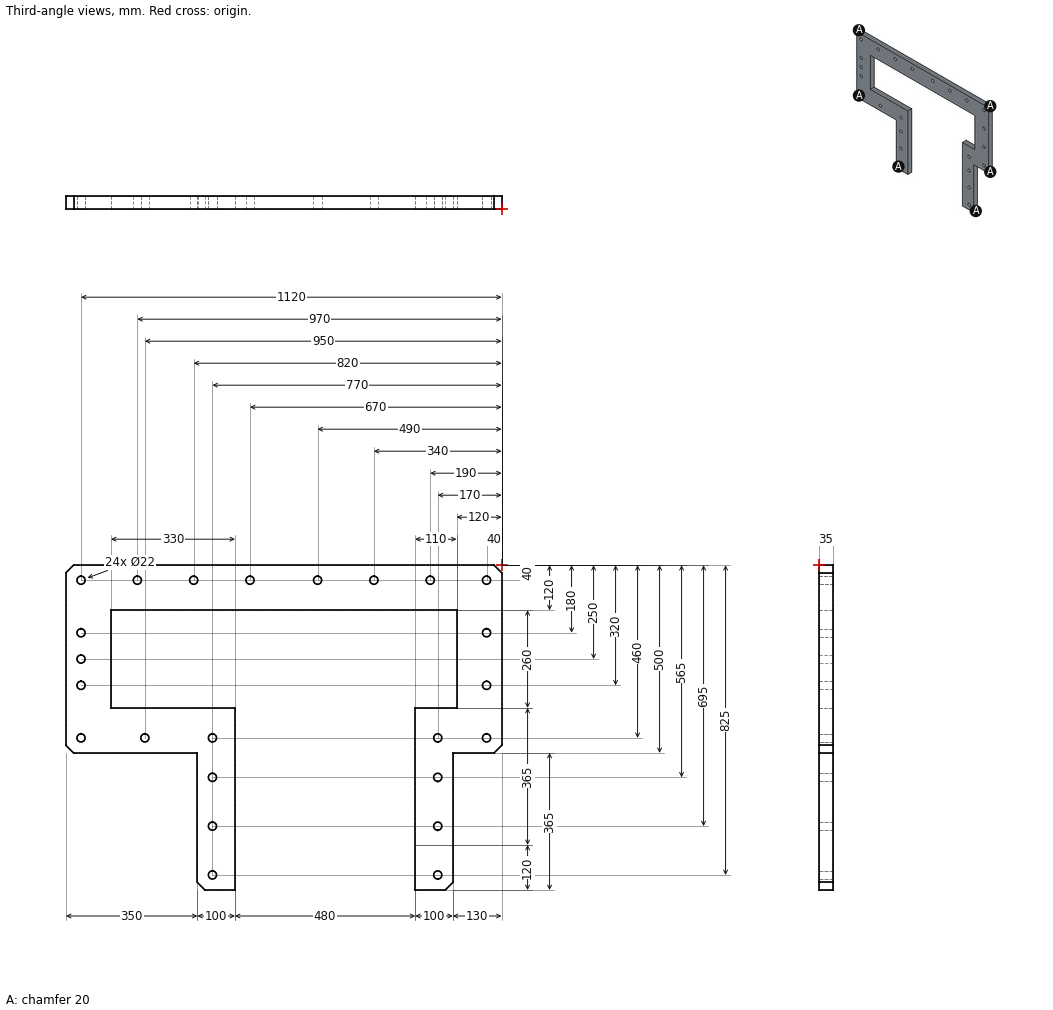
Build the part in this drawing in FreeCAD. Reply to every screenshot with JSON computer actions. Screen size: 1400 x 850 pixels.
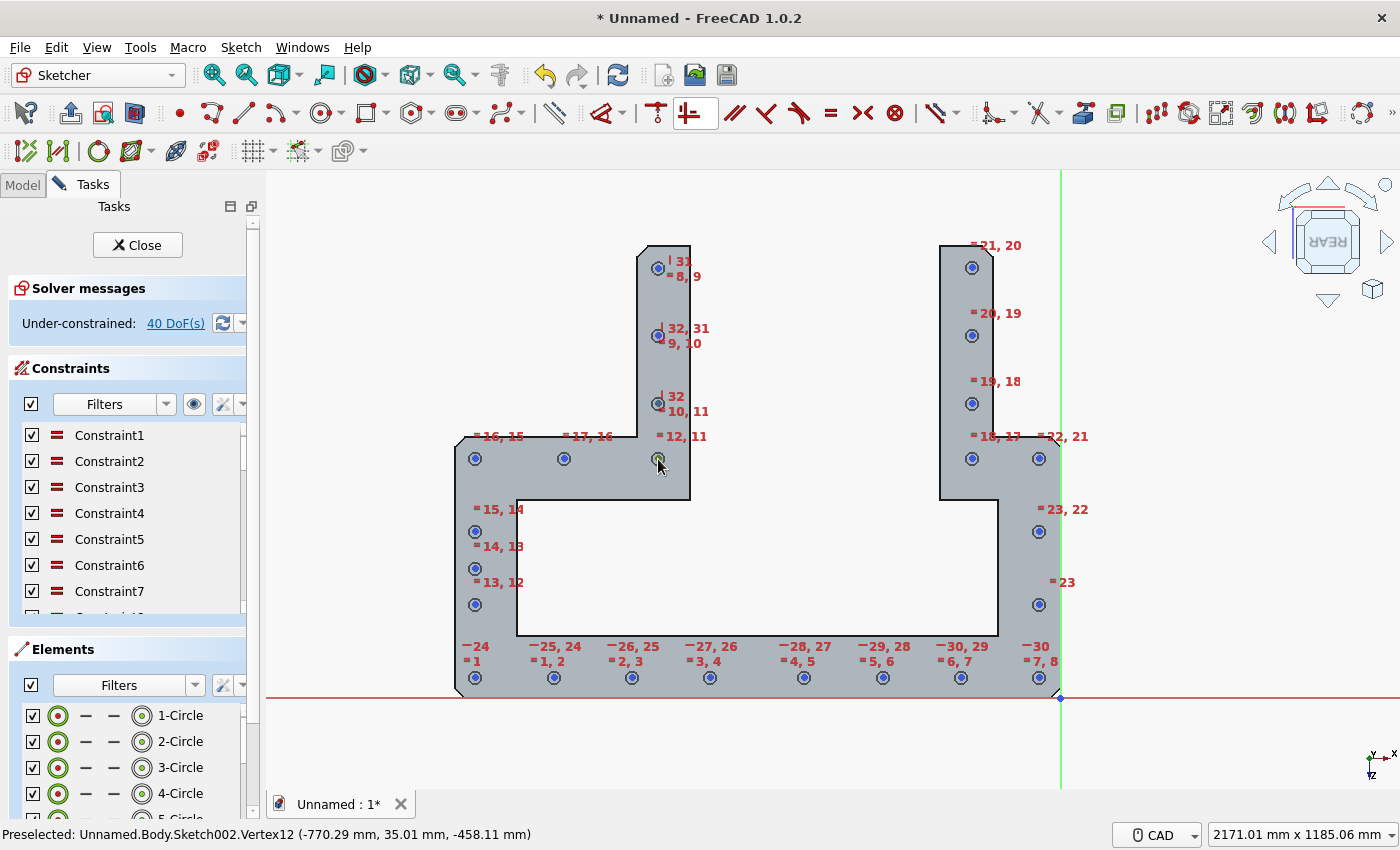
{"action": "left_click", "coordinate": [712, 114]}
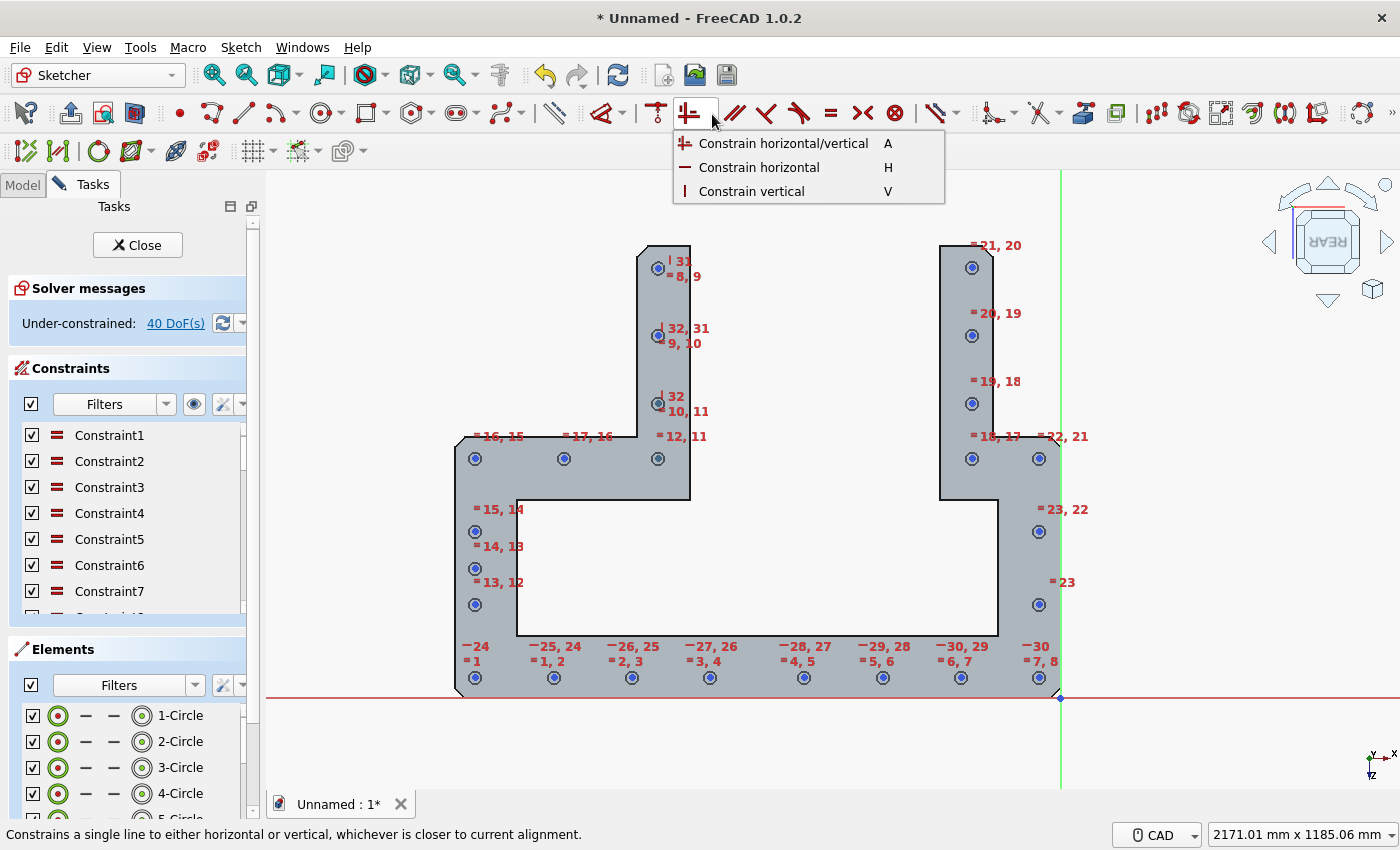
{"action": "left_click", "coordinate": [809, 191]}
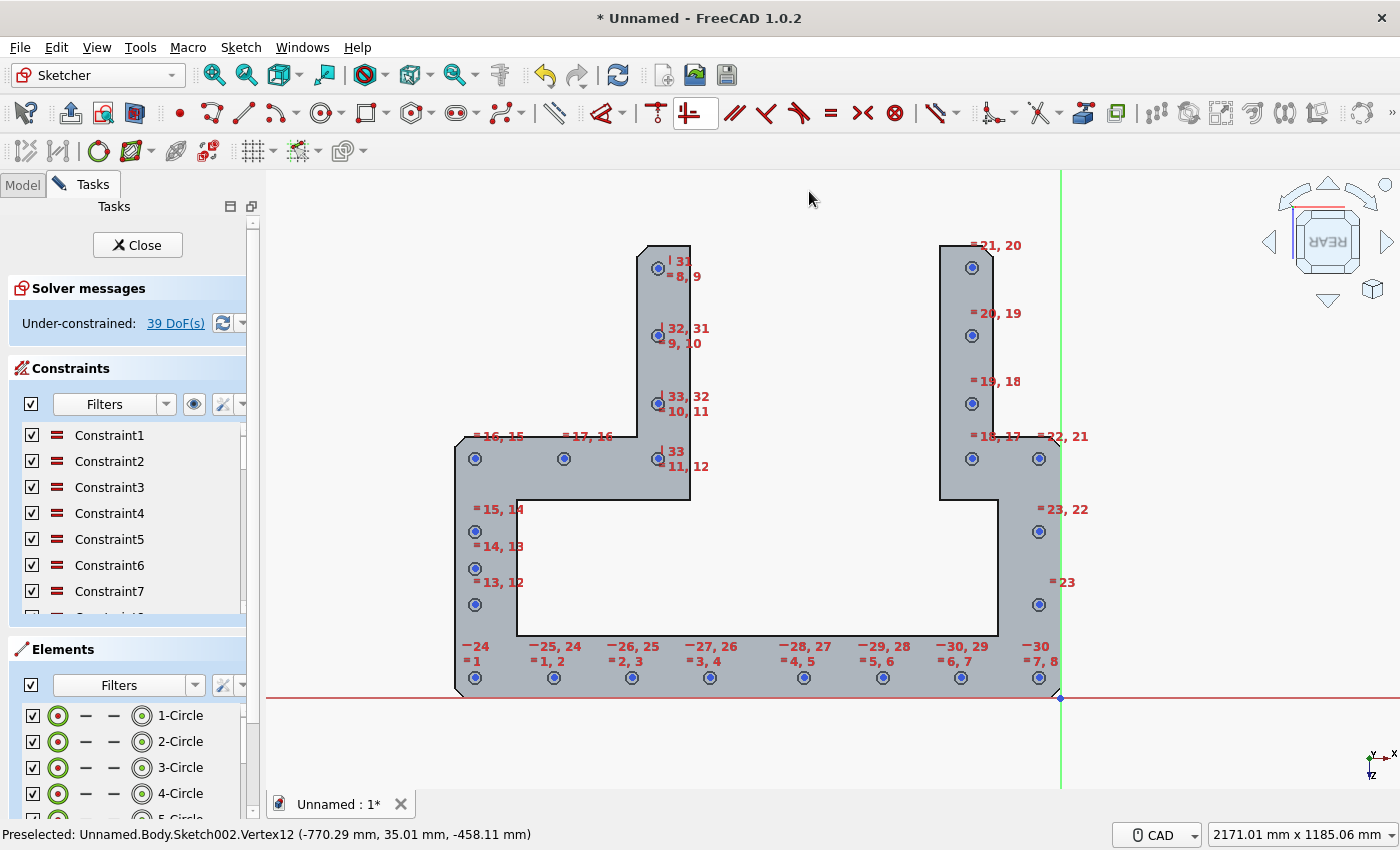
{"action": "left_click", "coordinate": [475, 678]}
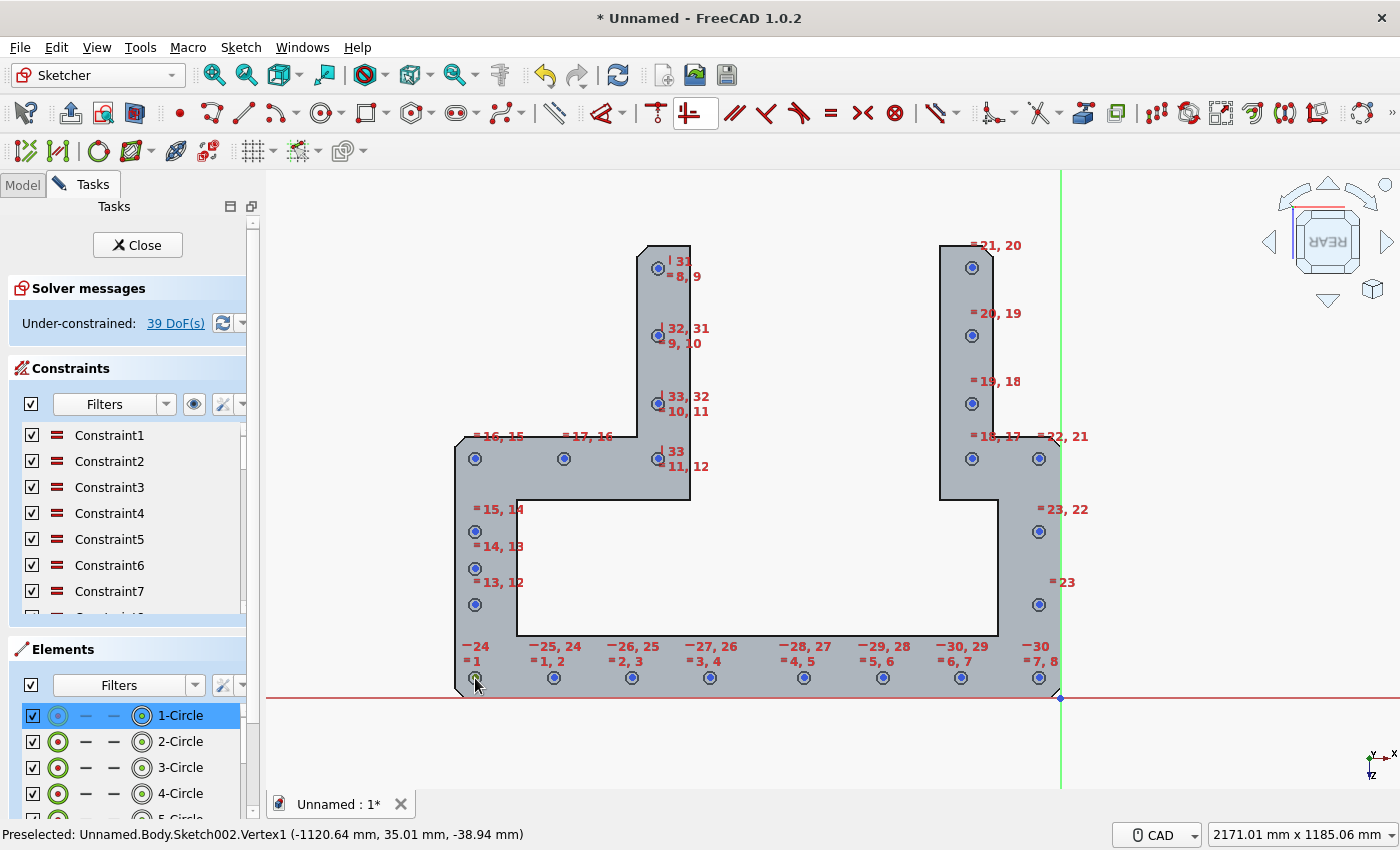
{"action": "left_click", "coordinate": [475, 605]}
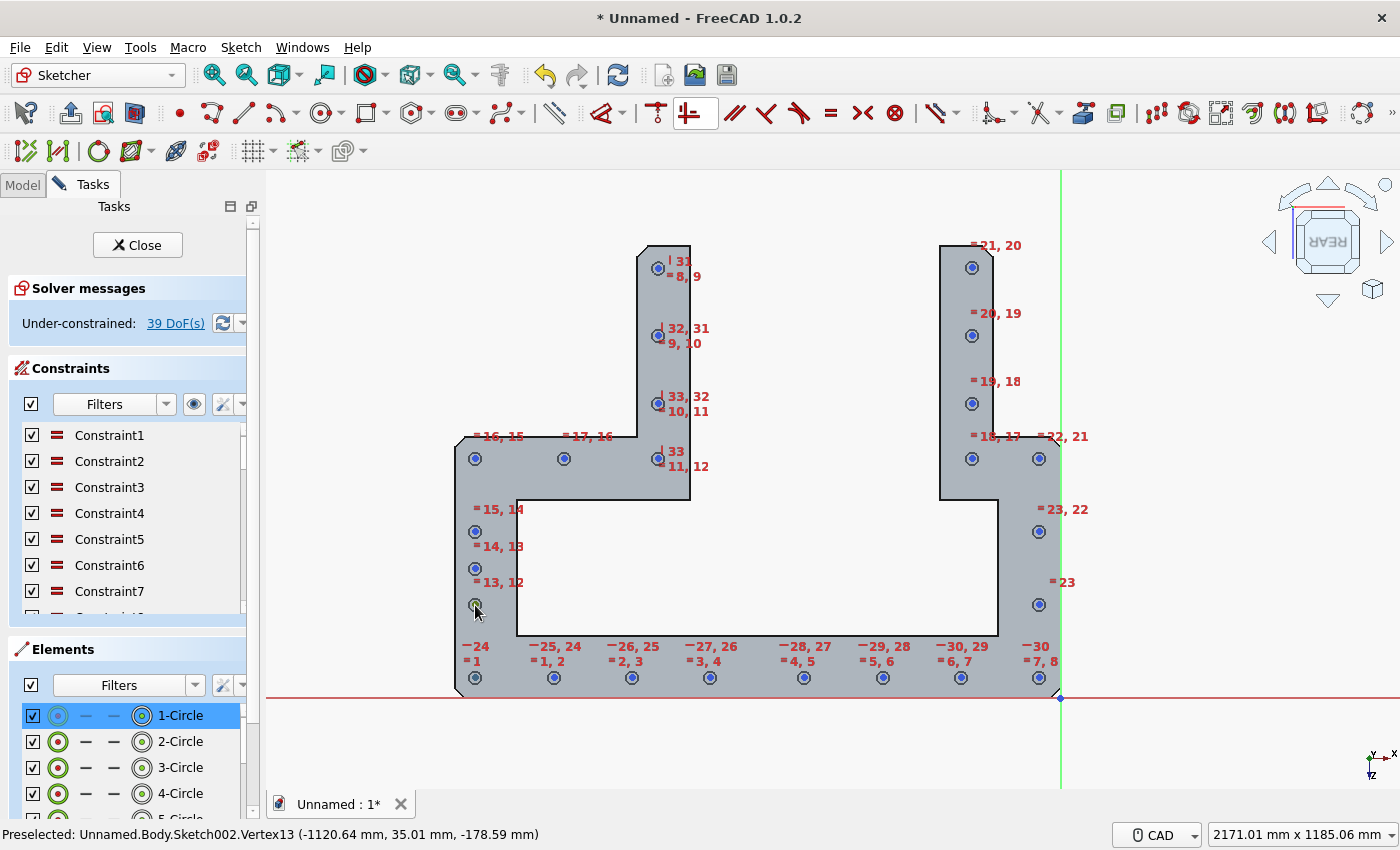
{"action": "key", "text": "v"}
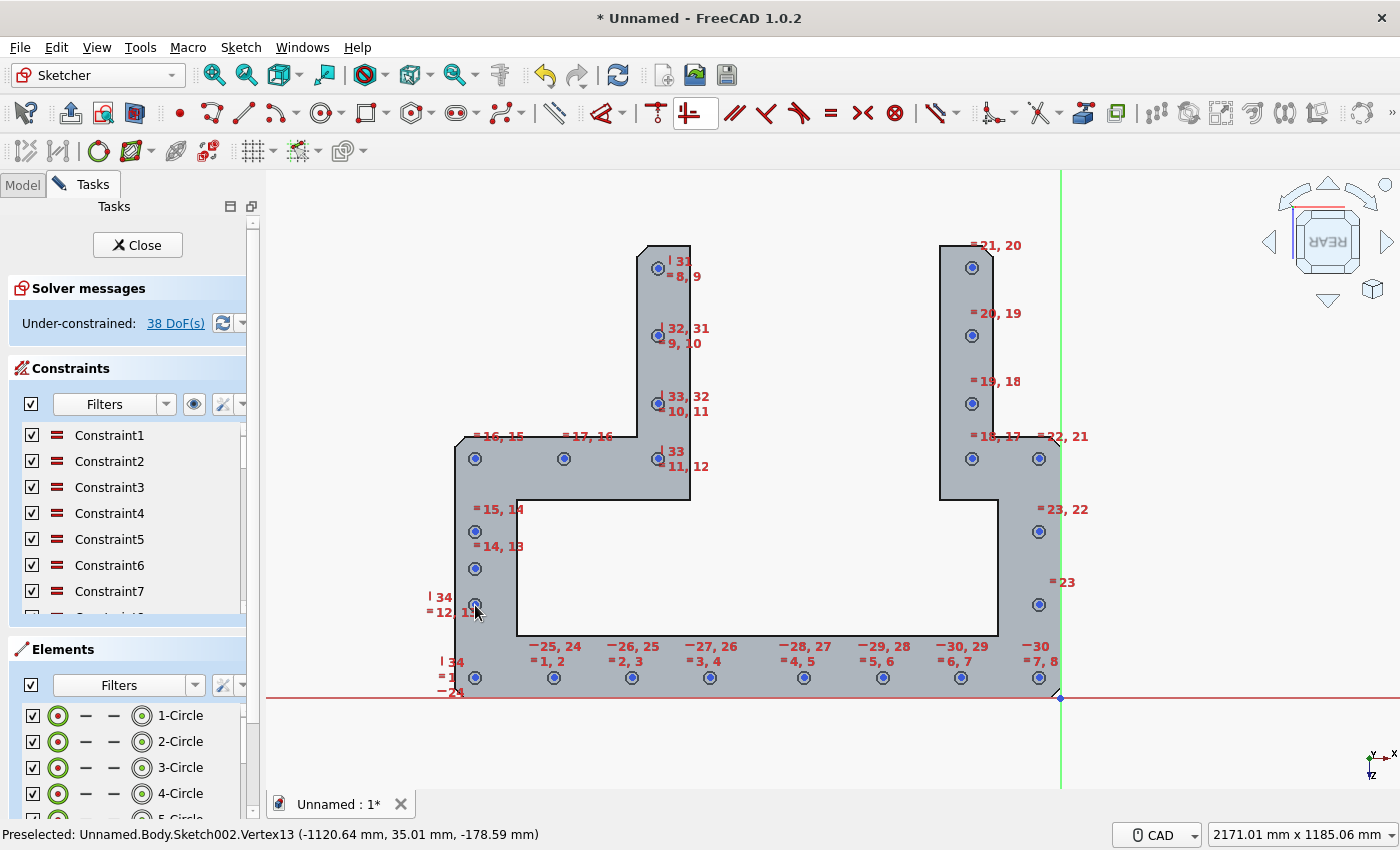
{"action": "left_click", "coordinate": [477, 607]}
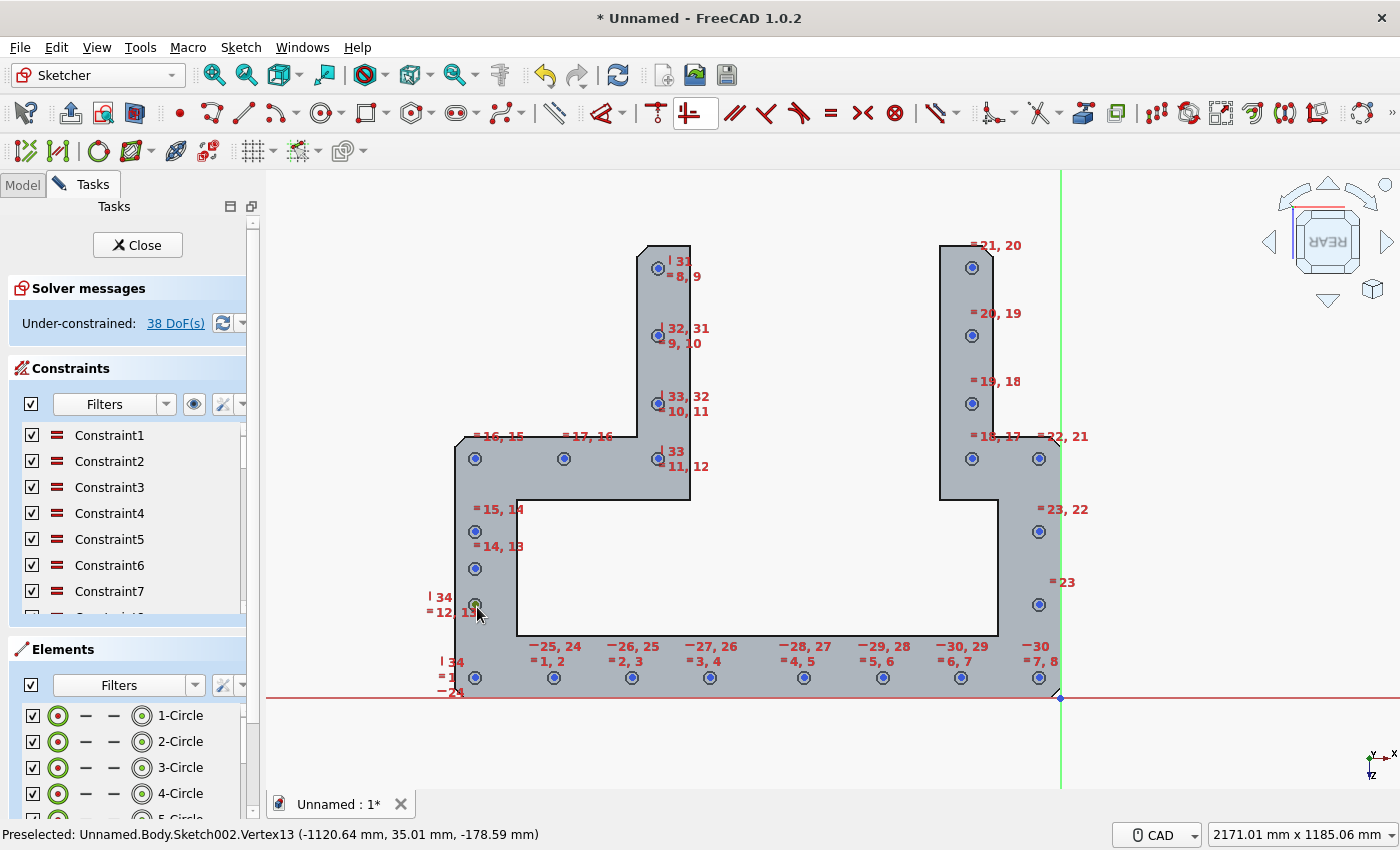
{"action": "left_click", "coordinate": [475, 569]}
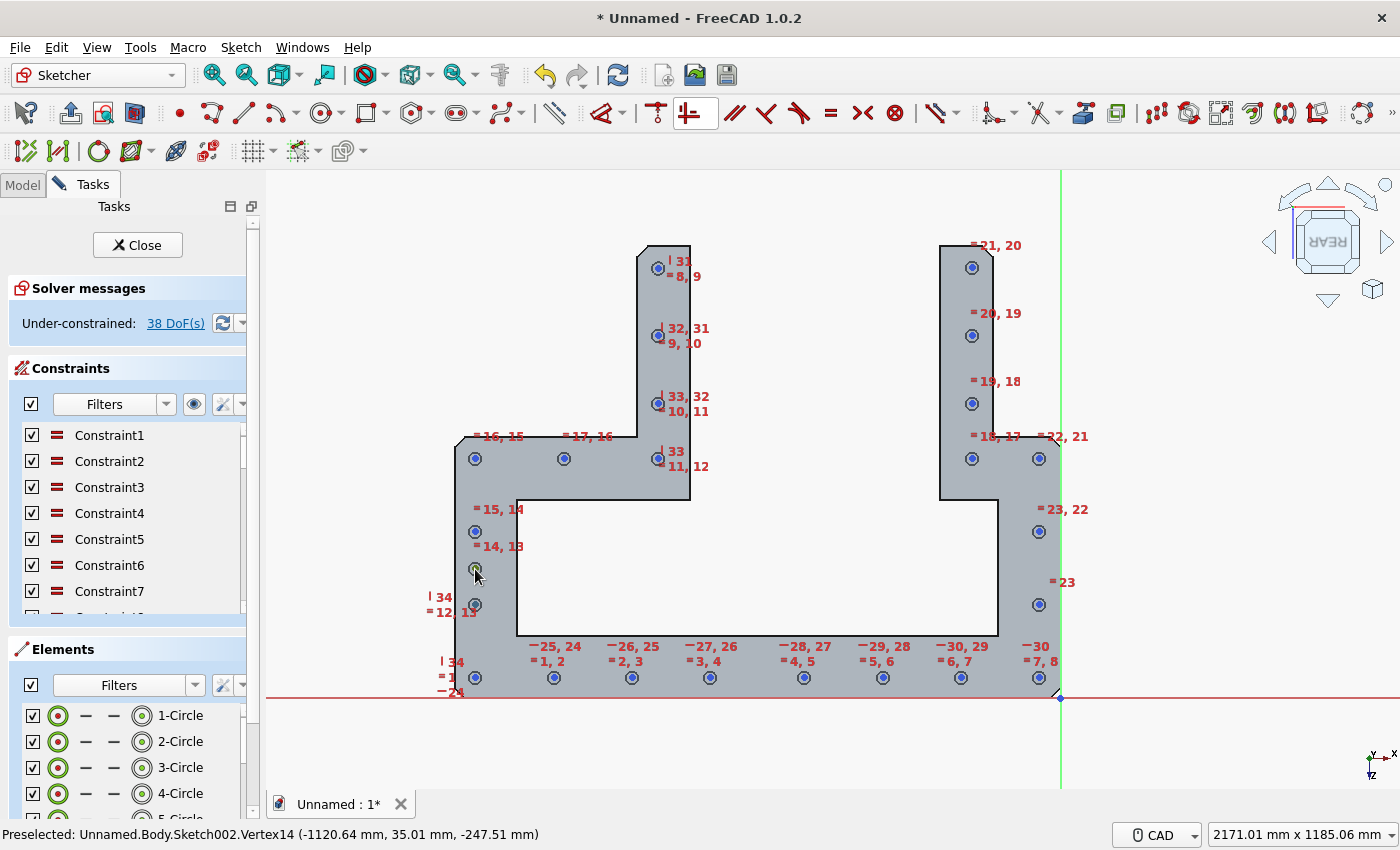
{"action": "key", "text": "v"}